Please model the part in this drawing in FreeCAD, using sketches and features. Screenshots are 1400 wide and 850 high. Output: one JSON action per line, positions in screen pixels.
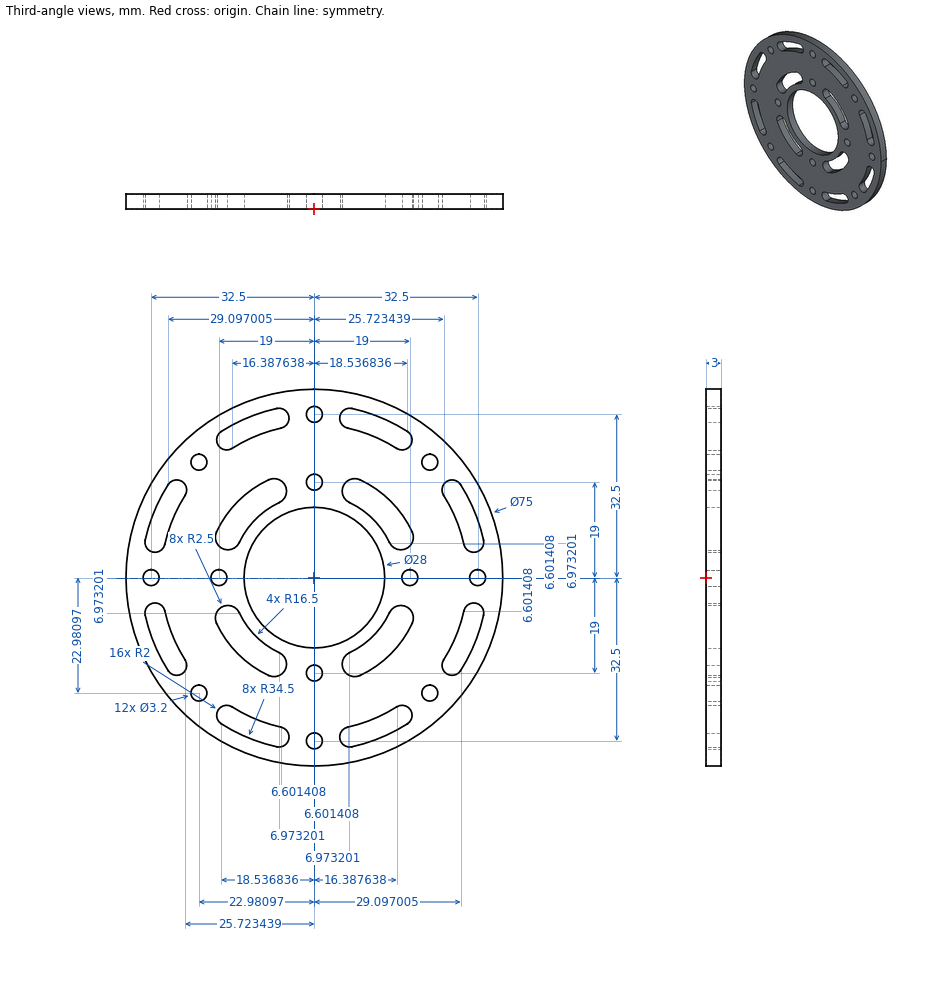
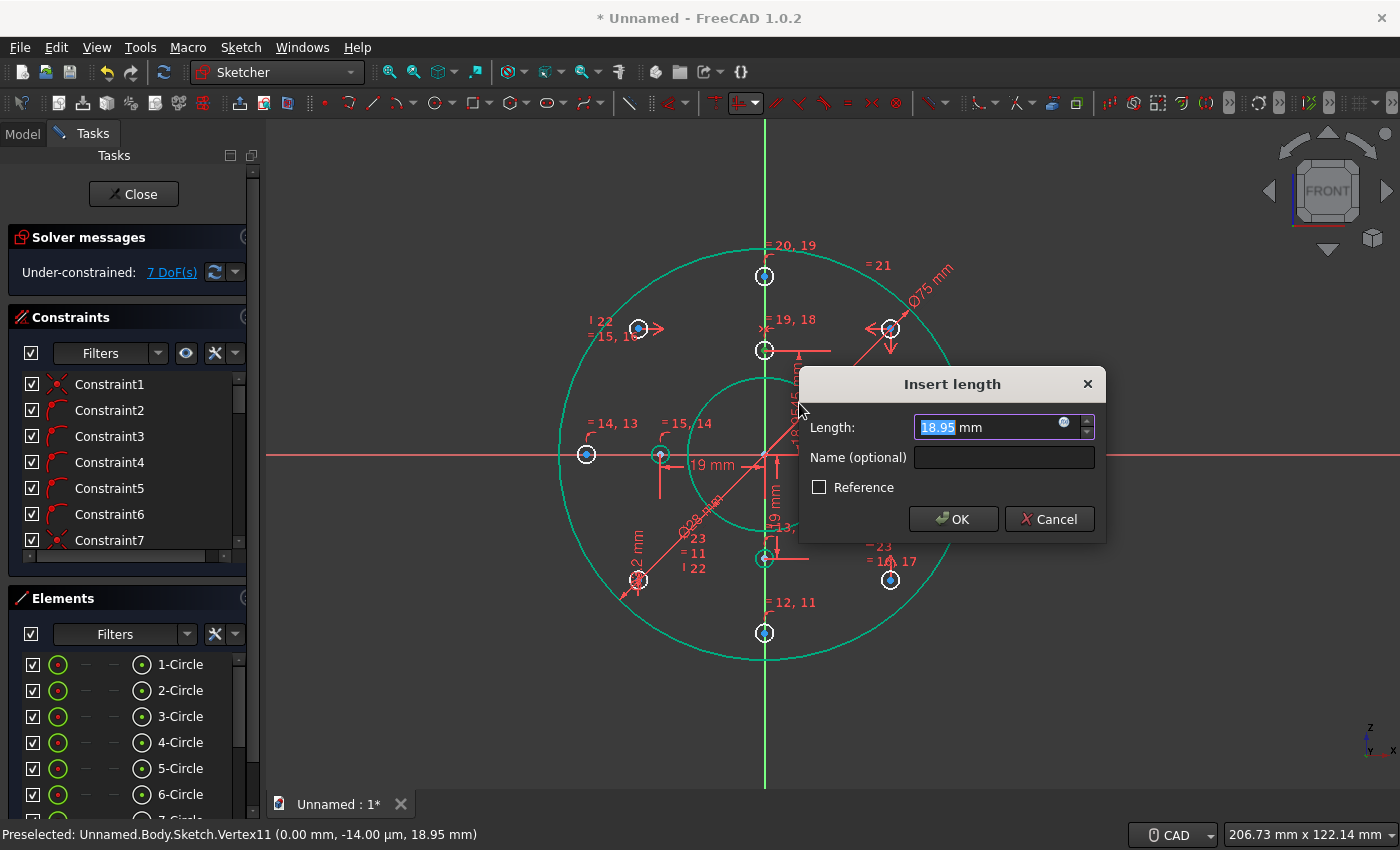
{"action": "type", "text": "19"}
{"action": "key", "text": "Return"}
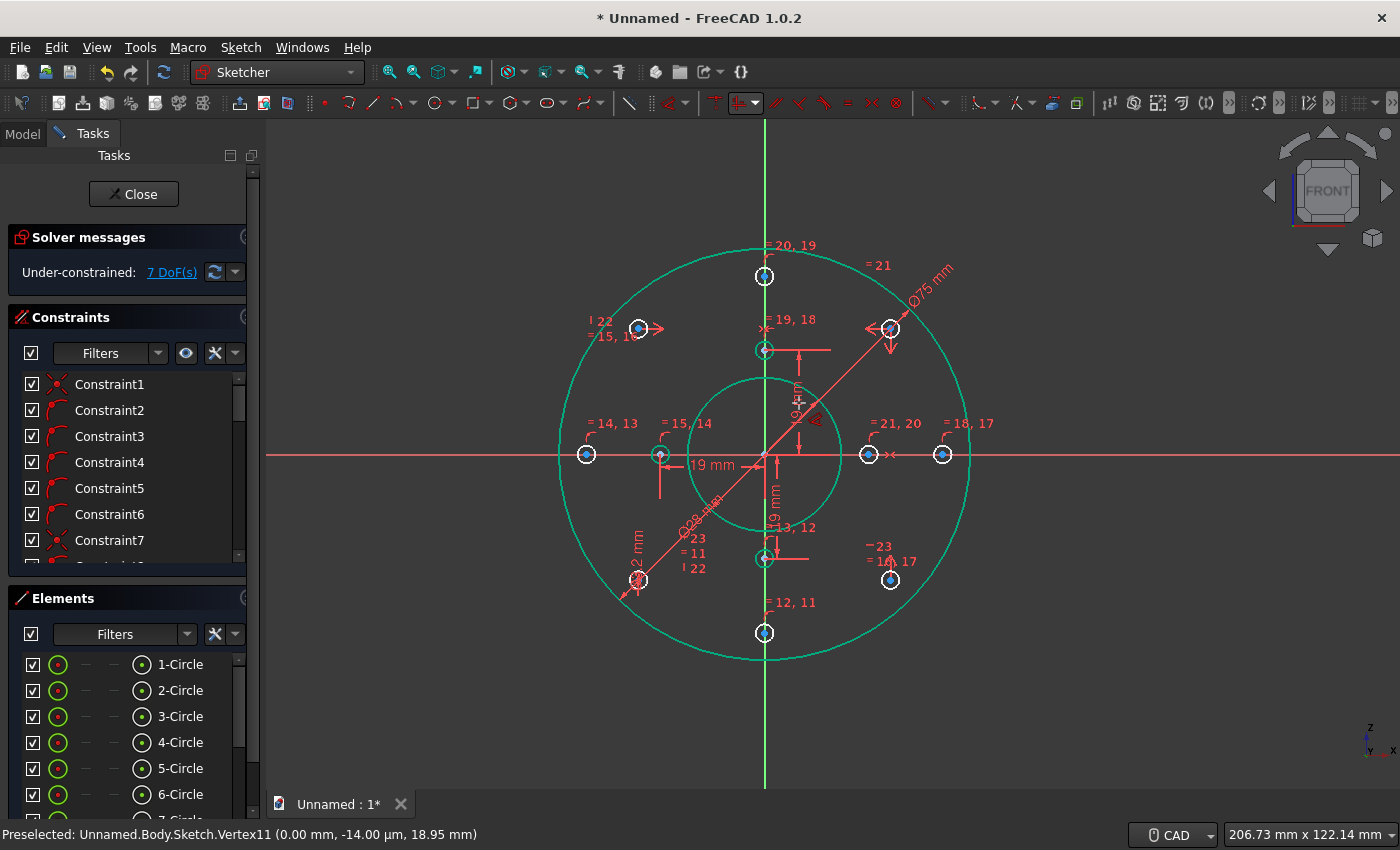
{"action": "left_click", "coordinate": [869, 455]}
{"action": "left_click", "coordinate": [853, 489]}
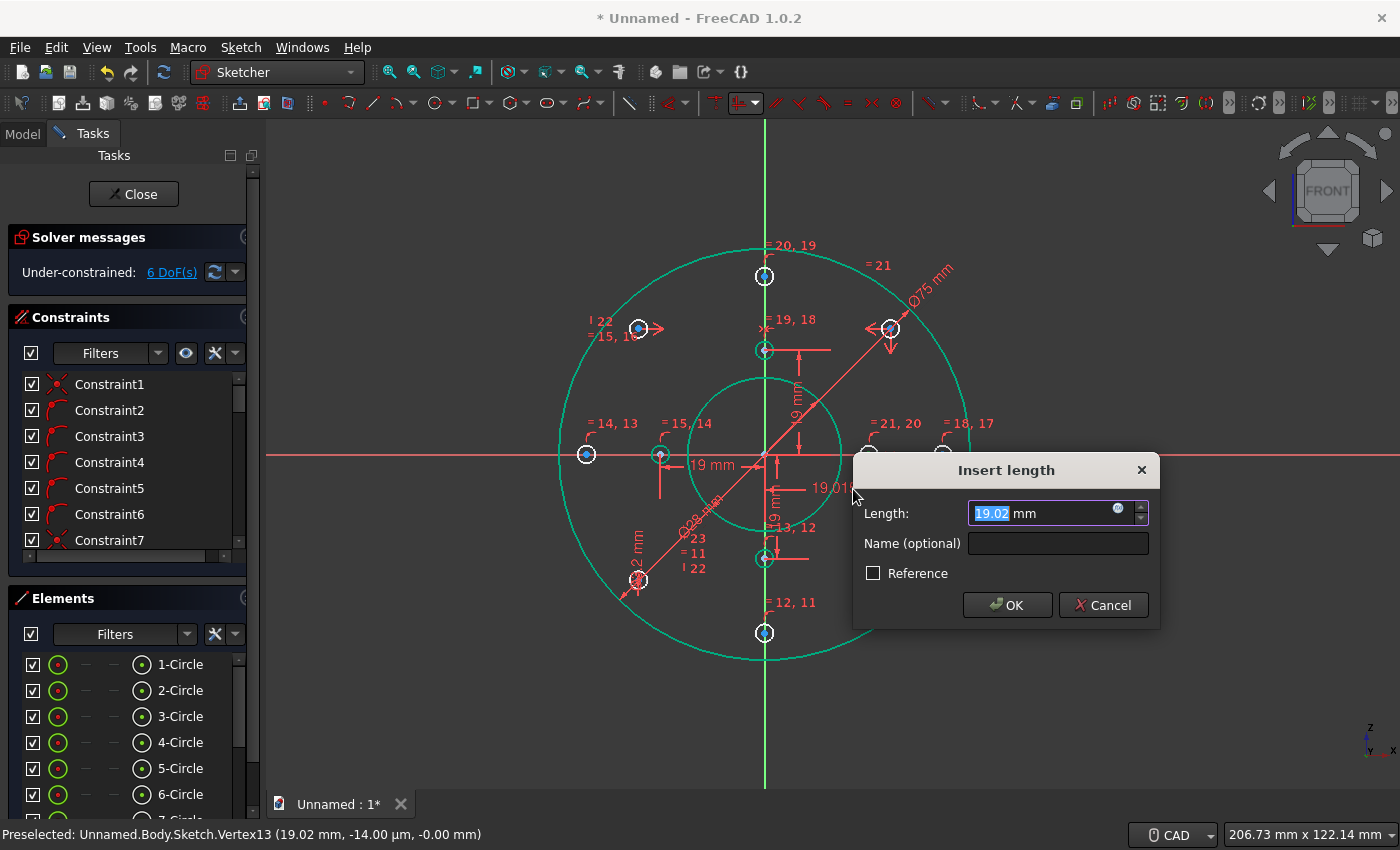
{"action": "type", "text": "19"}
{"action": "key", "text": "Return"}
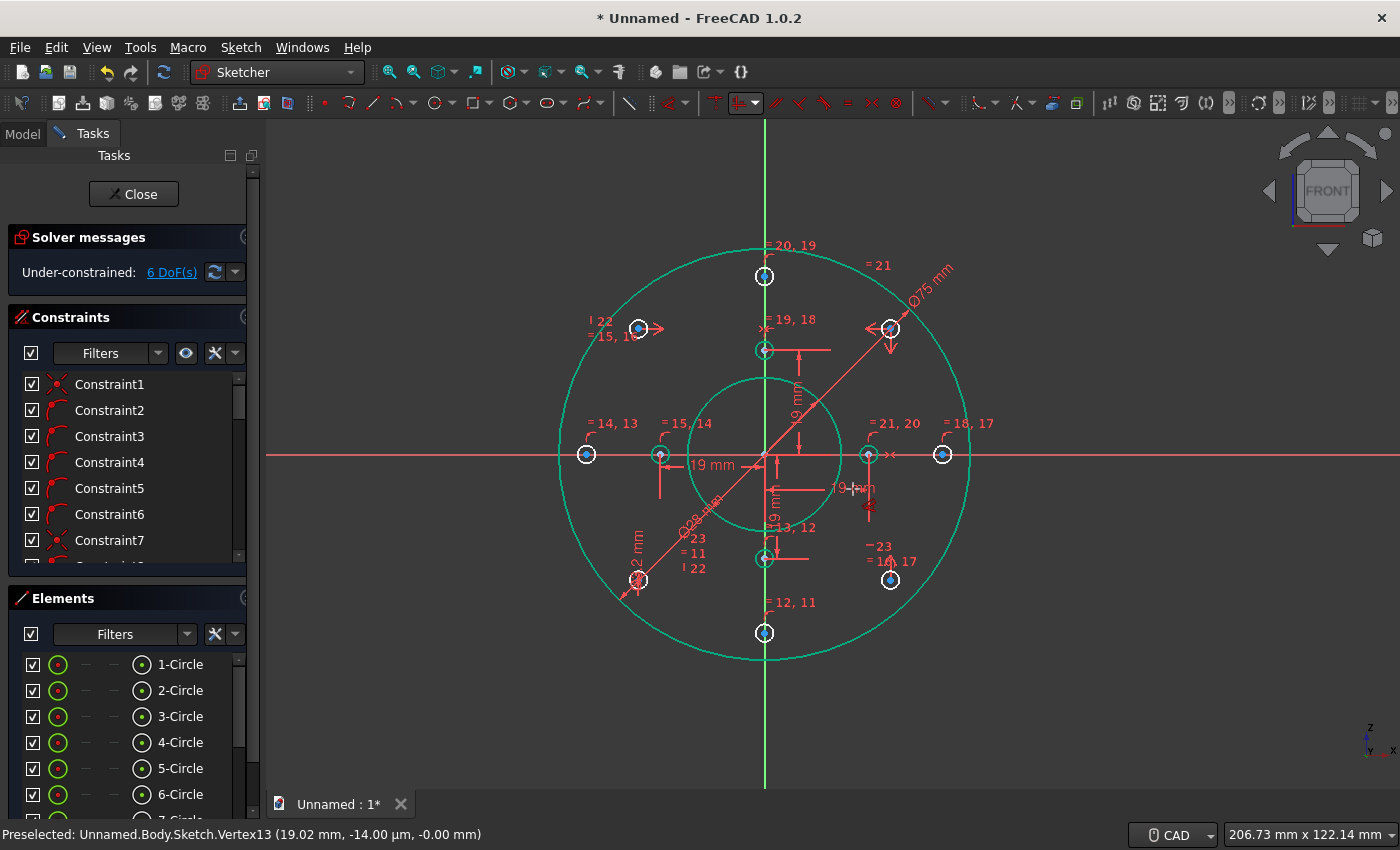
{"action": "left_click", "coordinate": [765, 633]}
{"action": "left_click", "coordinate": [799, 544]}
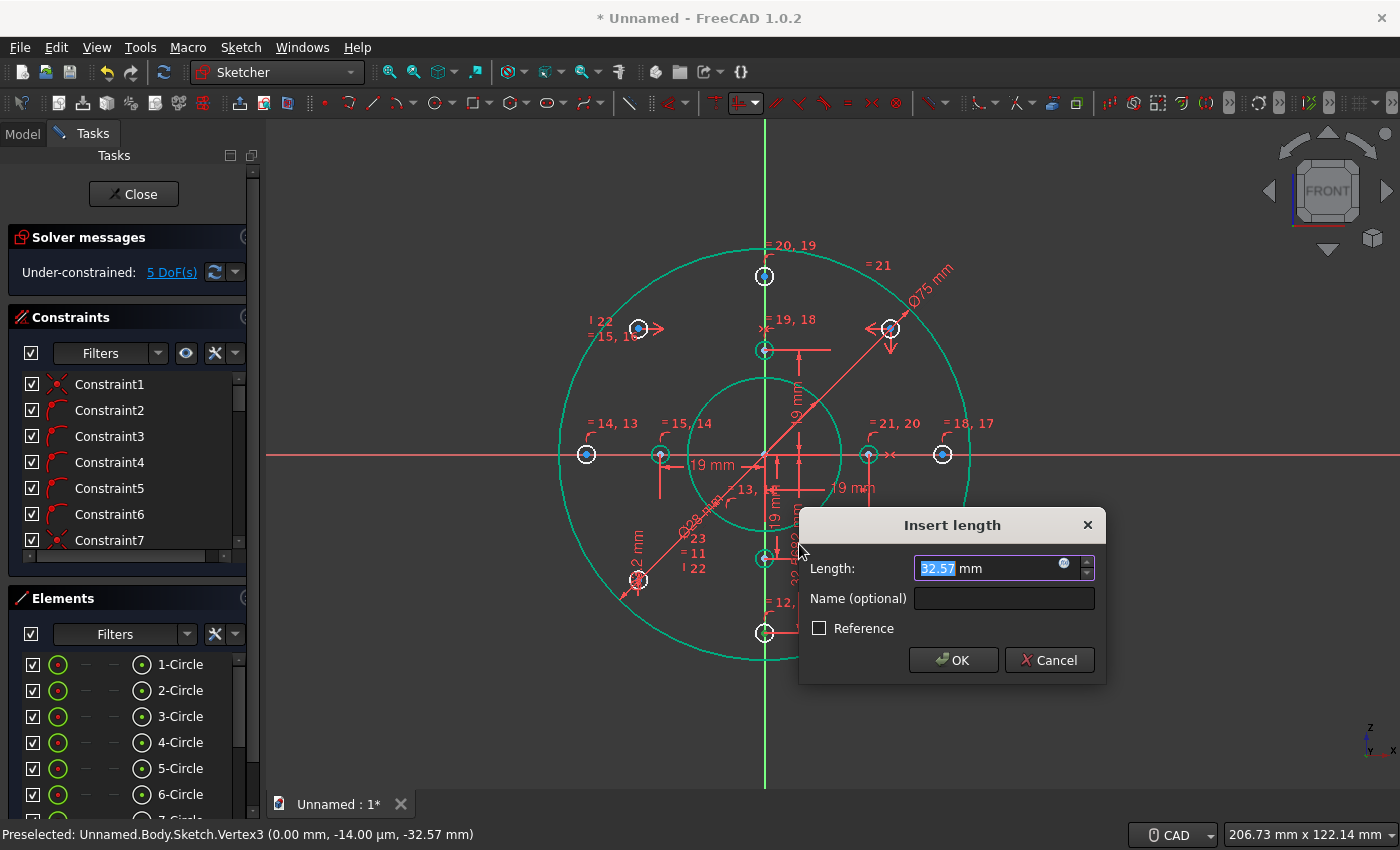
{"action": "type", "text": "32.5"}
{"action": "key", "text": "Return"}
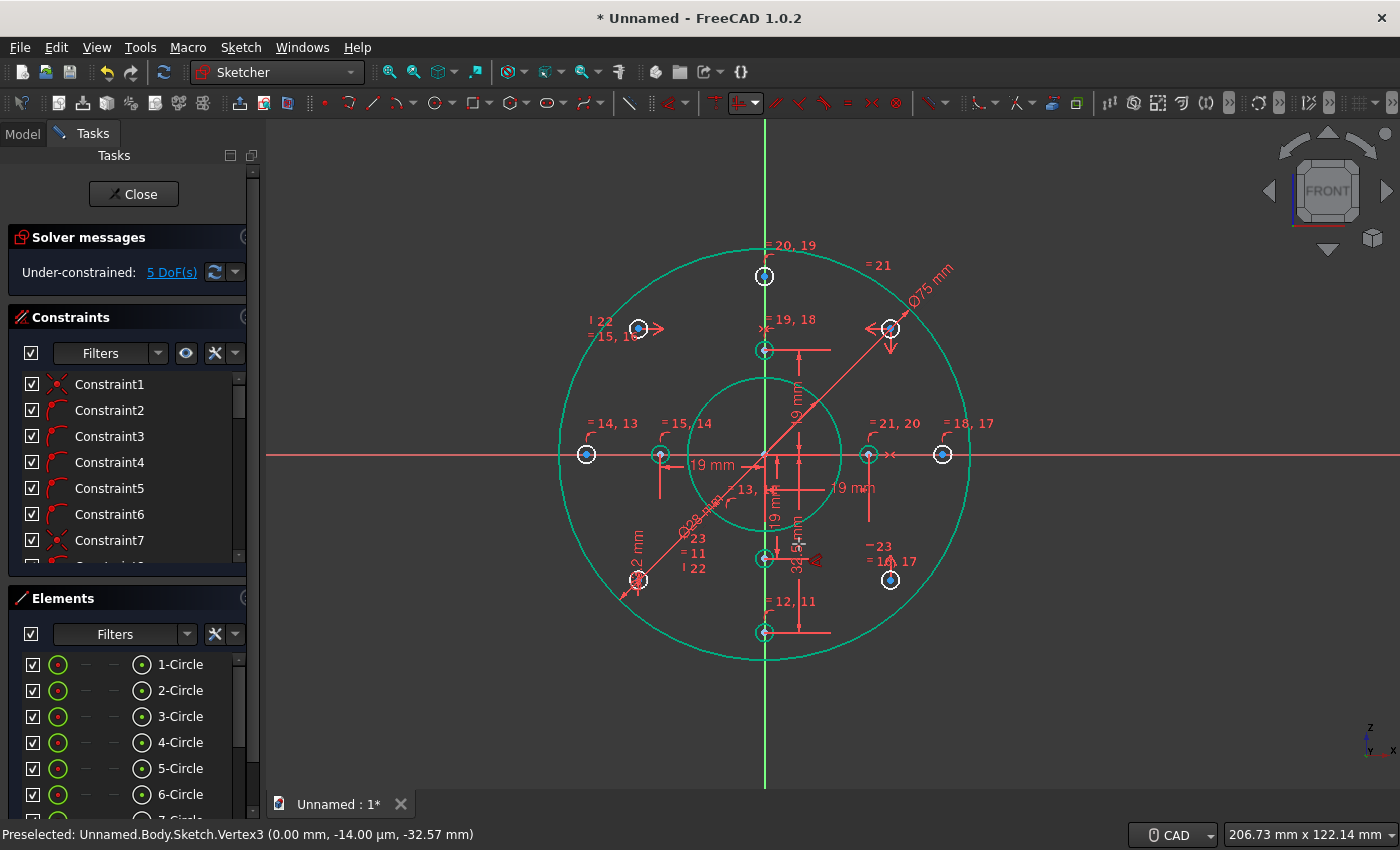
{"action": "left_click", "coordinate": [586, 455]}
{"action": "left_click", "coordinate": [675, 489]}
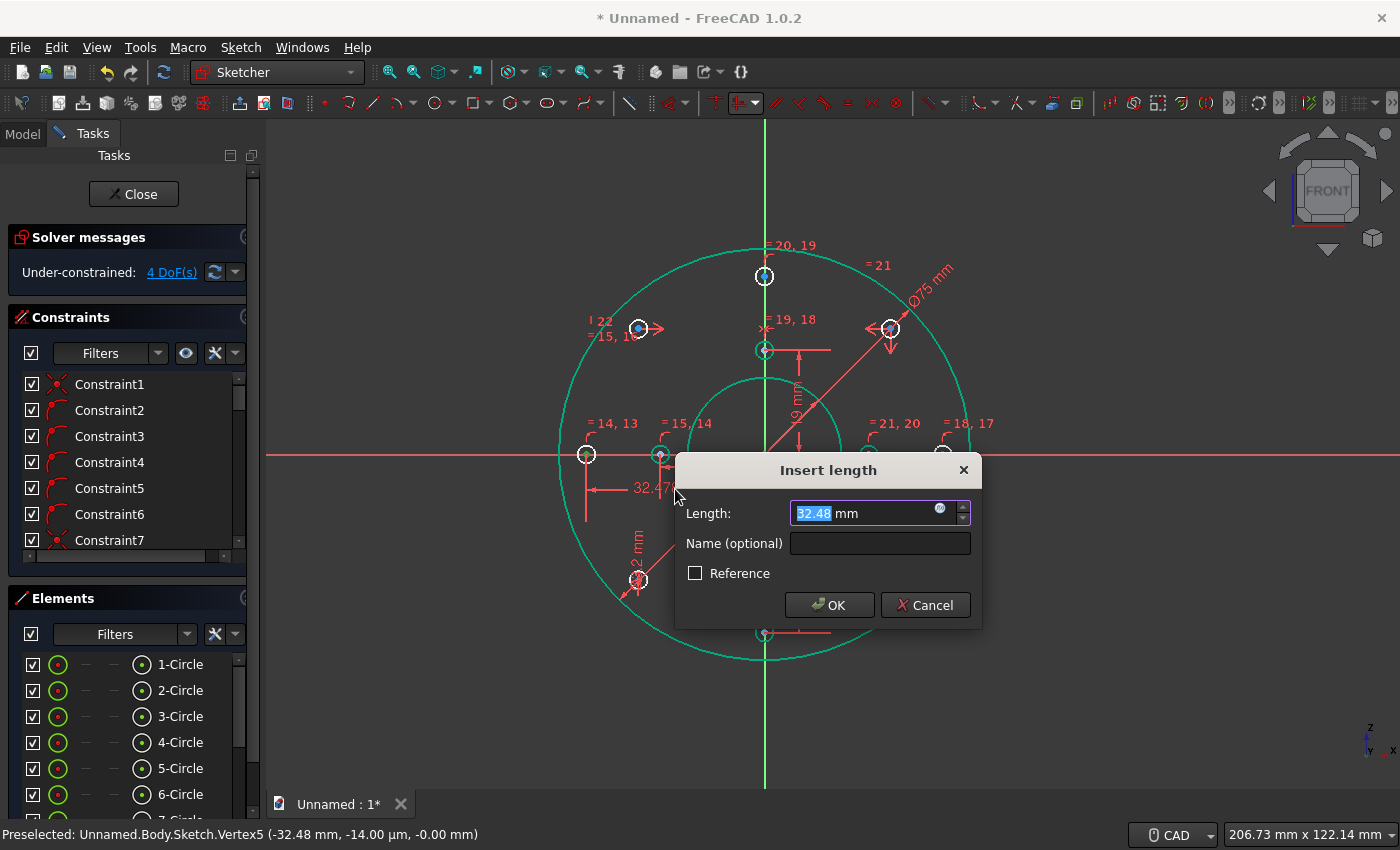
{"action": "type", "text": "32.5"}
{"action": "key", "text": "Return"}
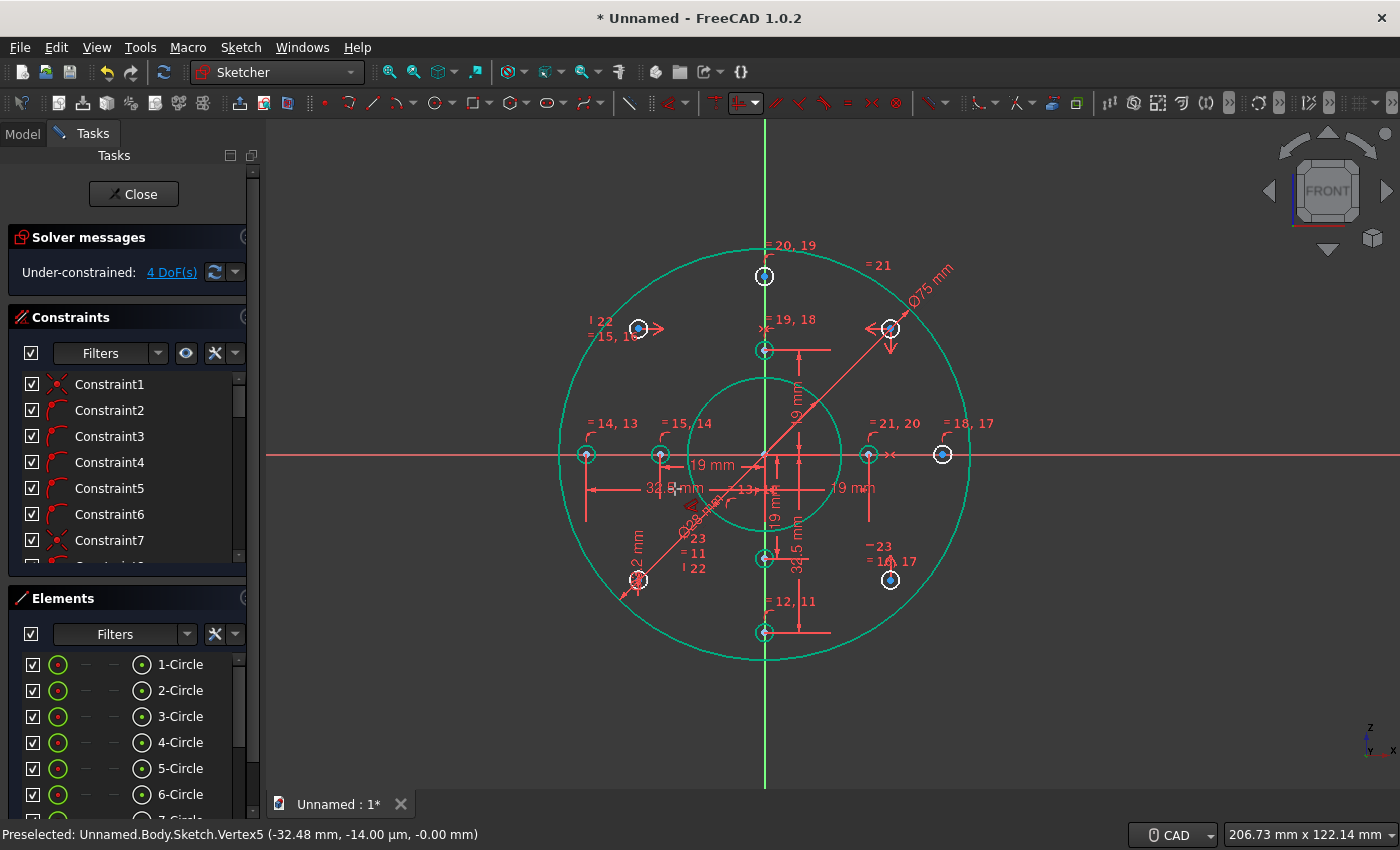
{"action": "left_click", "coordinate": [943, 455]}
{"action": "left_click", "coordinate": [895, 421]}